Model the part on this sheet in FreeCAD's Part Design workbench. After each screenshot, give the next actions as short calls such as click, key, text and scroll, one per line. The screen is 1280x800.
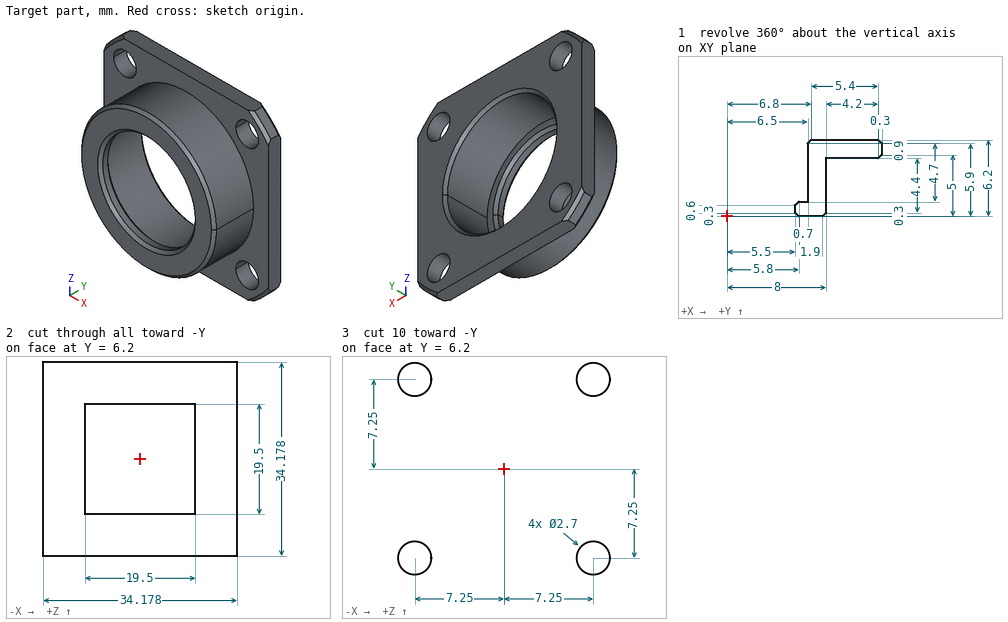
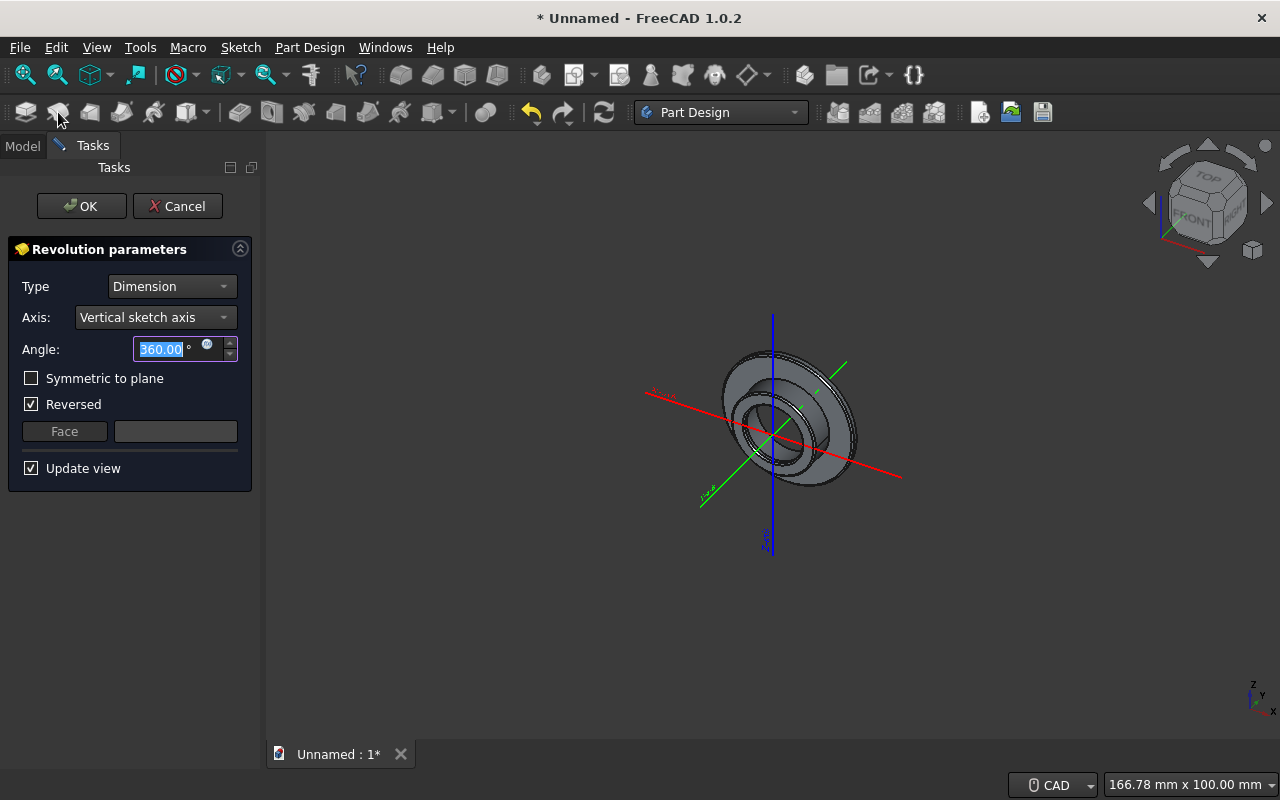
click(82, 206)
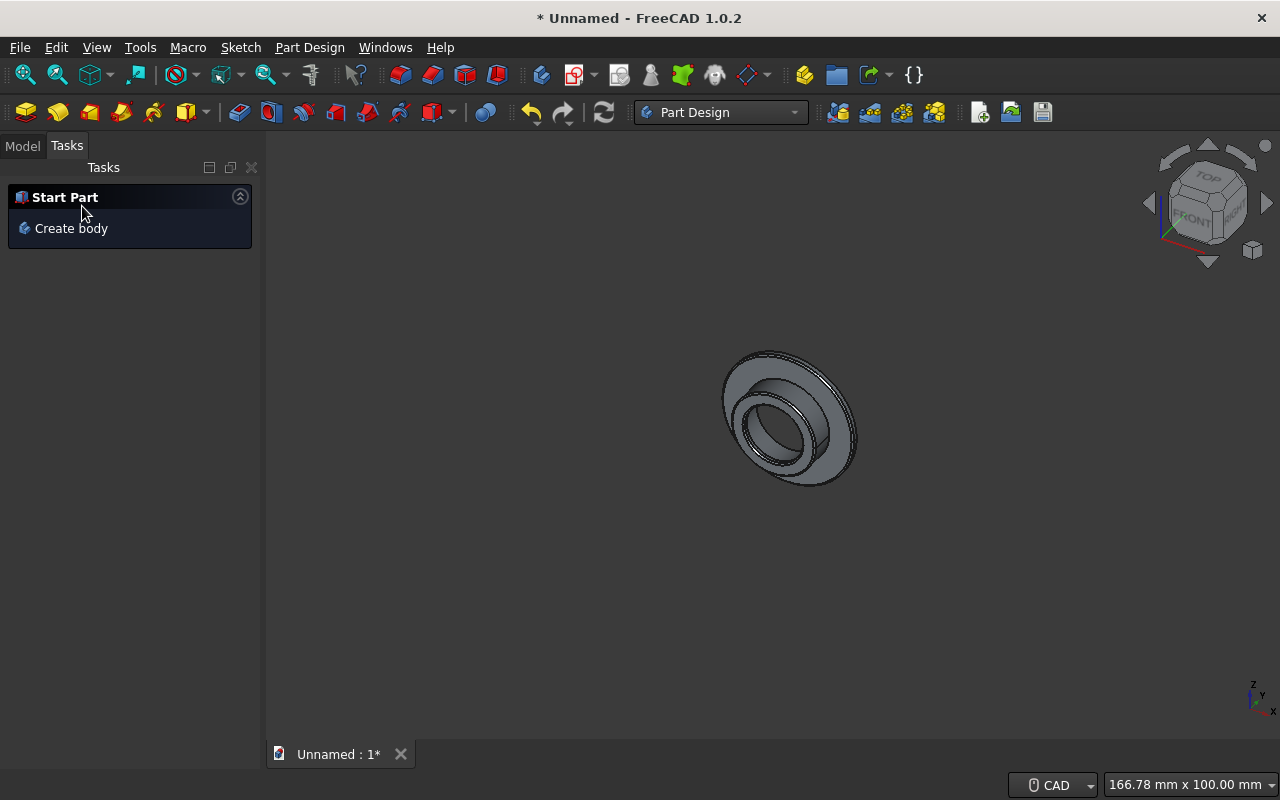
click(26, 76)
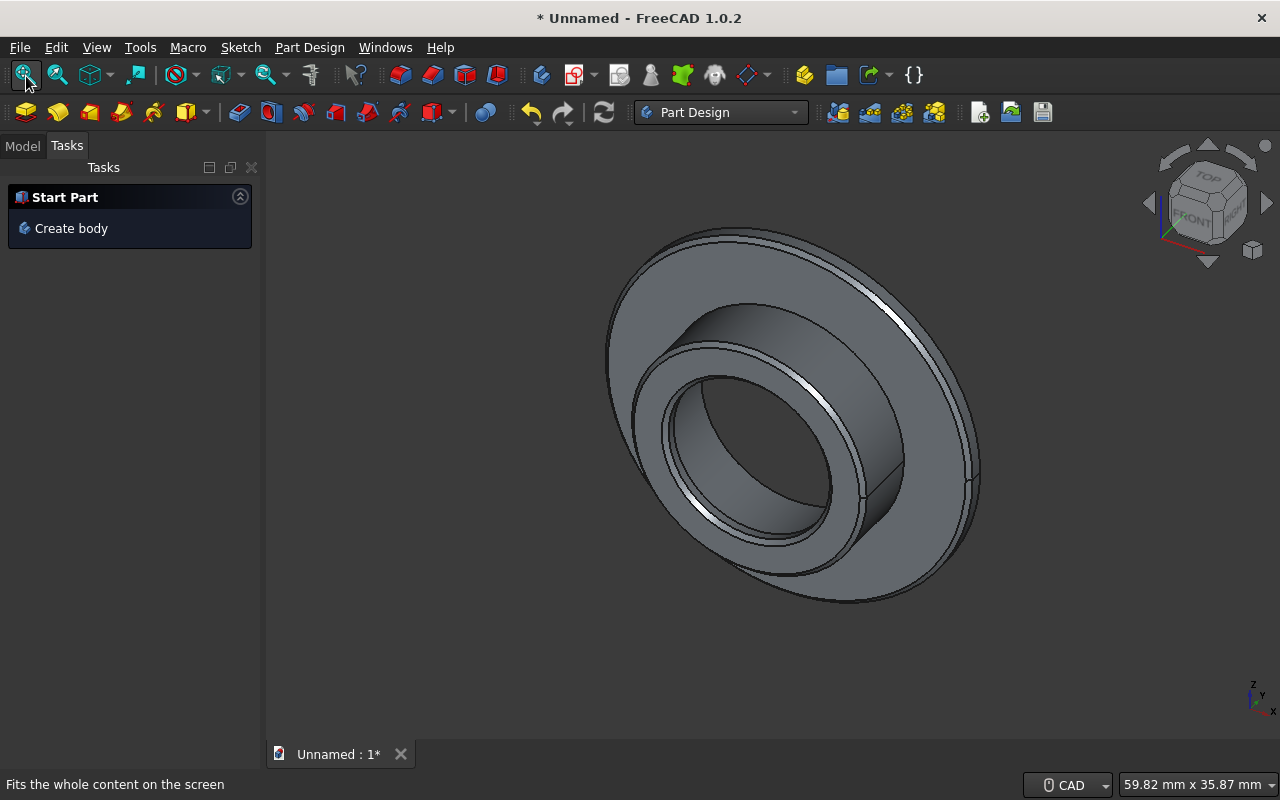
key(4)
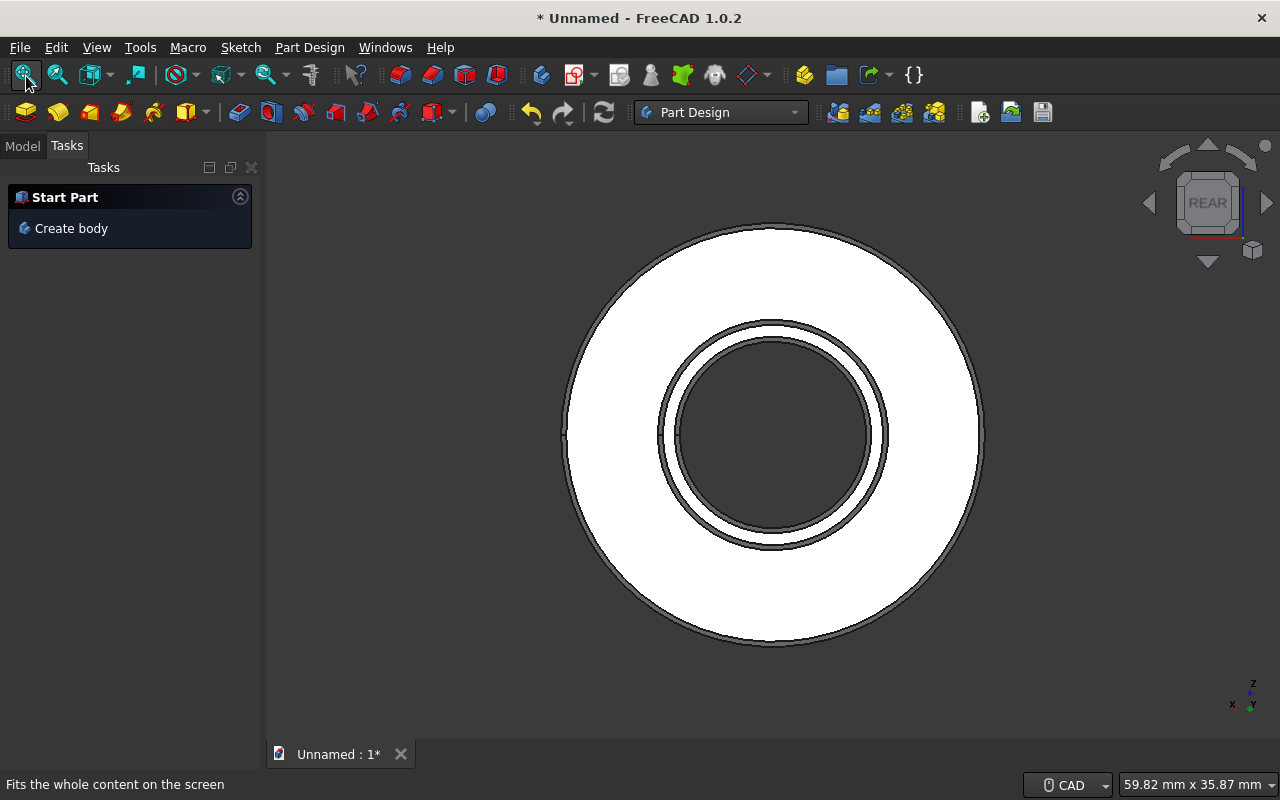
click(655, 316)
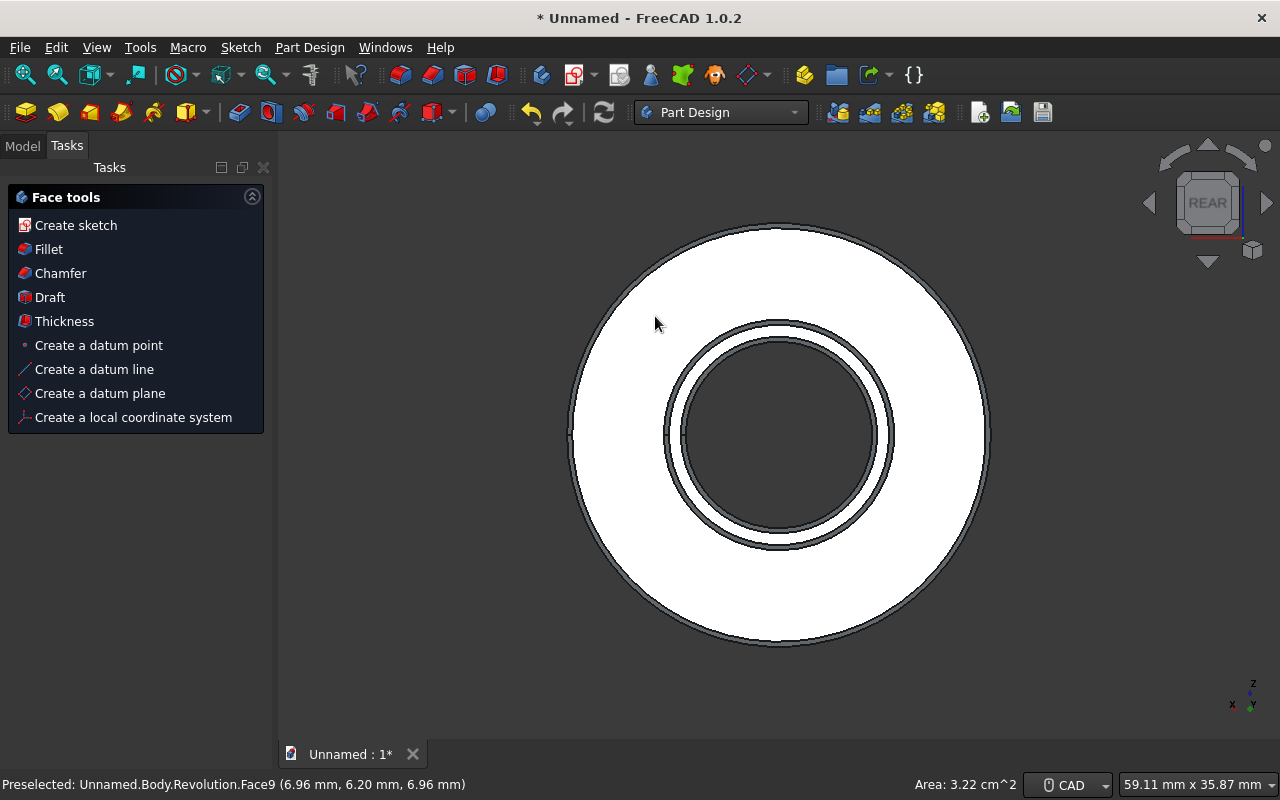
click(574, 76)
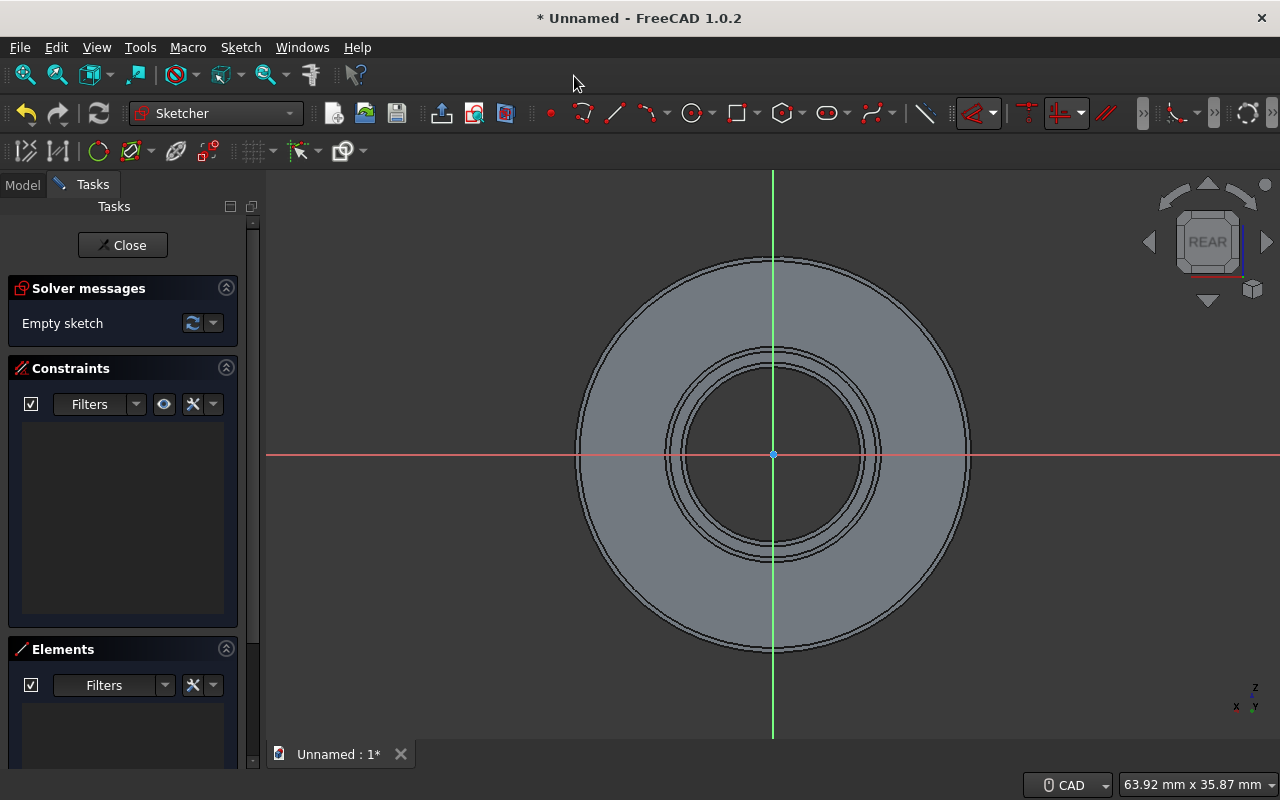
scroll(565, 455, down, 2)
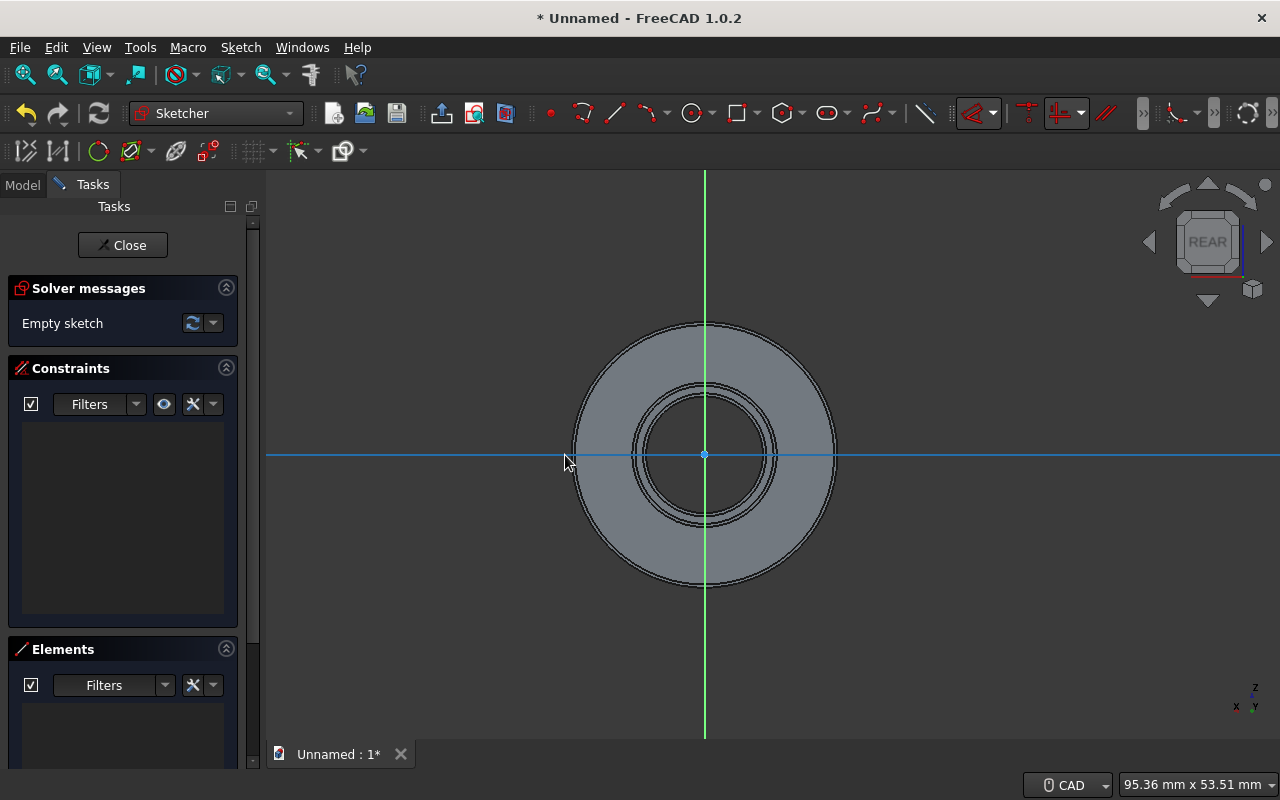
key(g)
key(v)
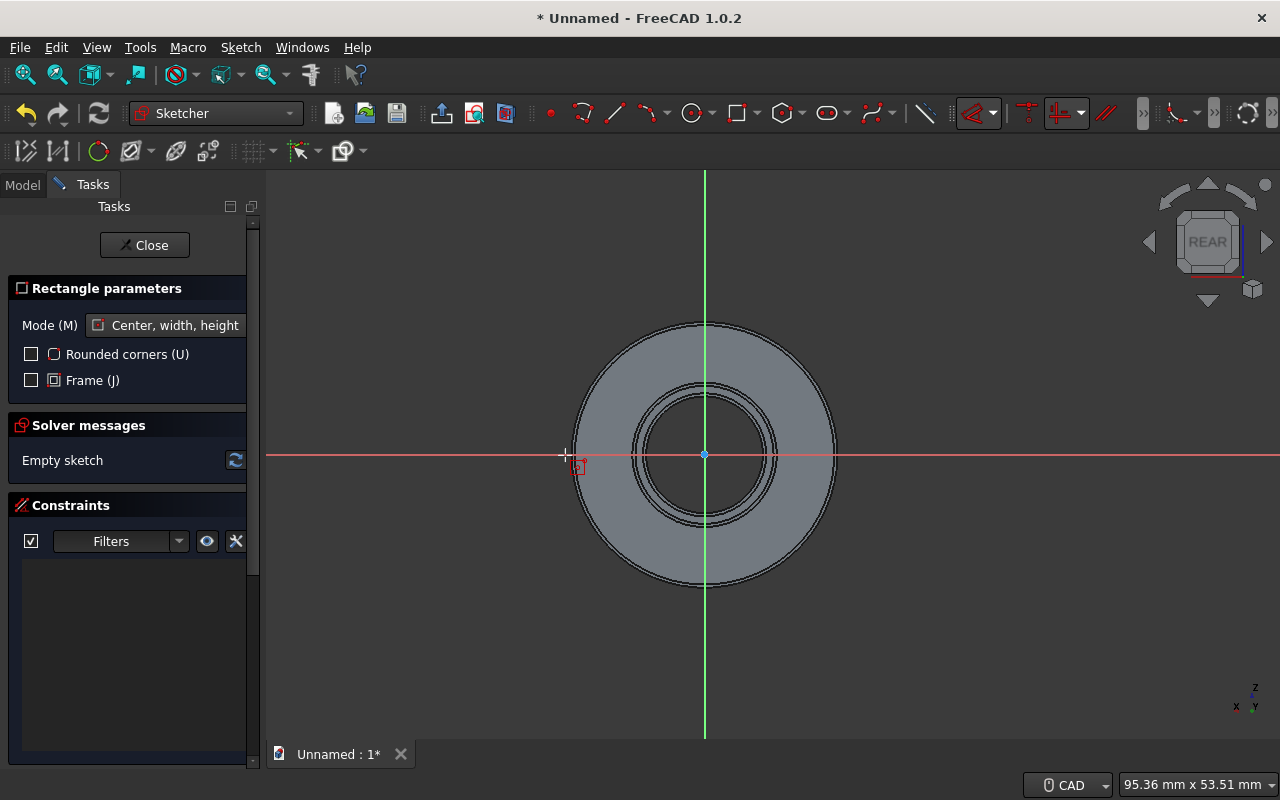
click(705, 455)
click(886, 273)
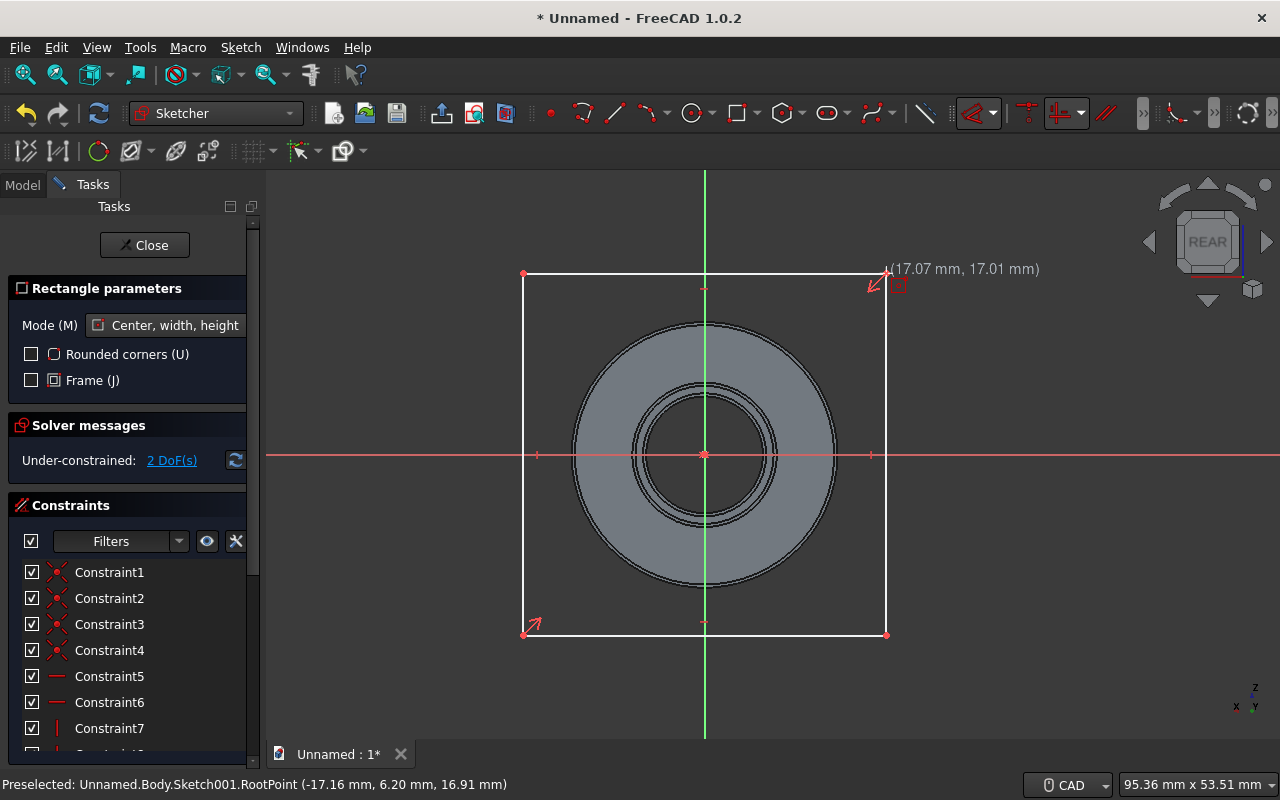
click(705, 455)
click(808, 351)
key(Escape)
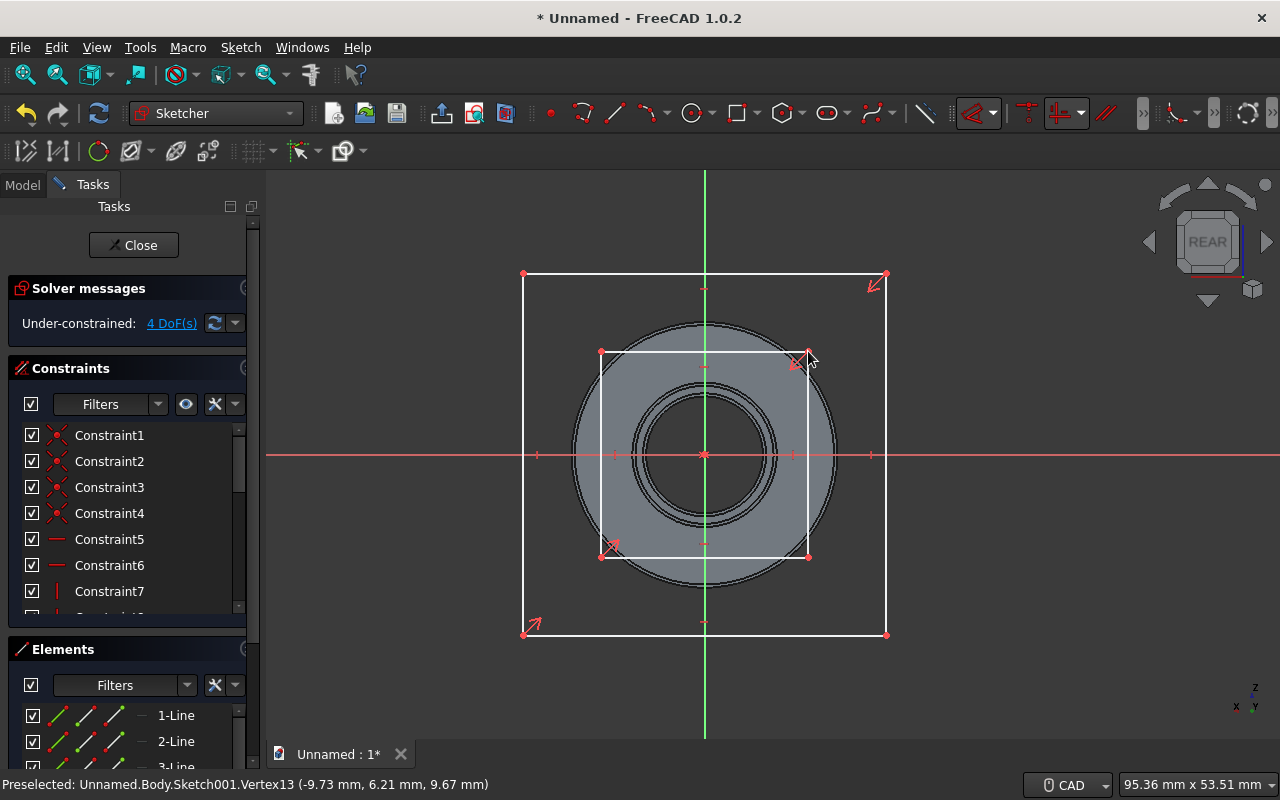
click(663, 558)